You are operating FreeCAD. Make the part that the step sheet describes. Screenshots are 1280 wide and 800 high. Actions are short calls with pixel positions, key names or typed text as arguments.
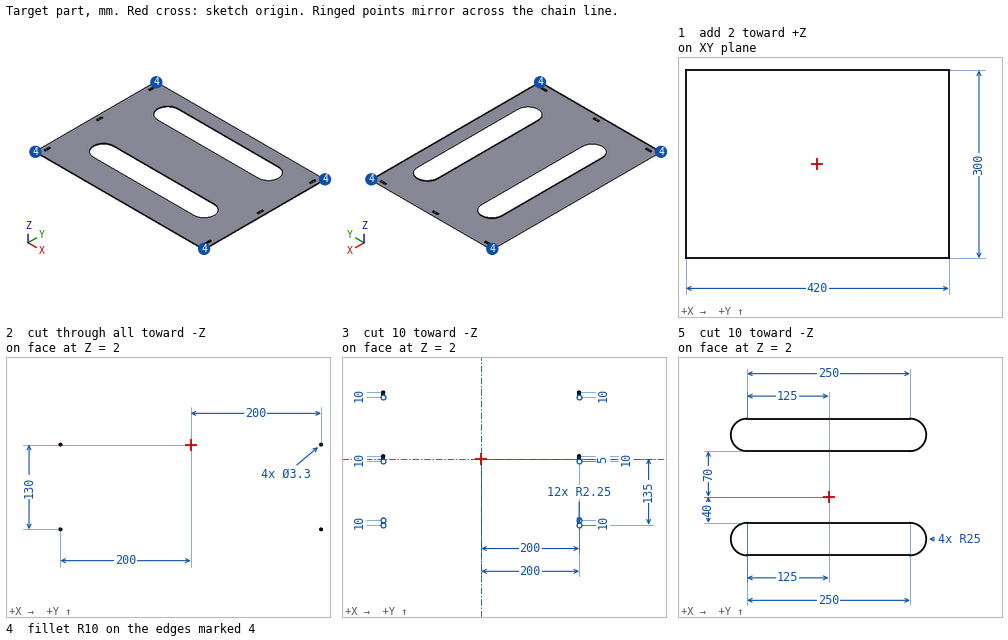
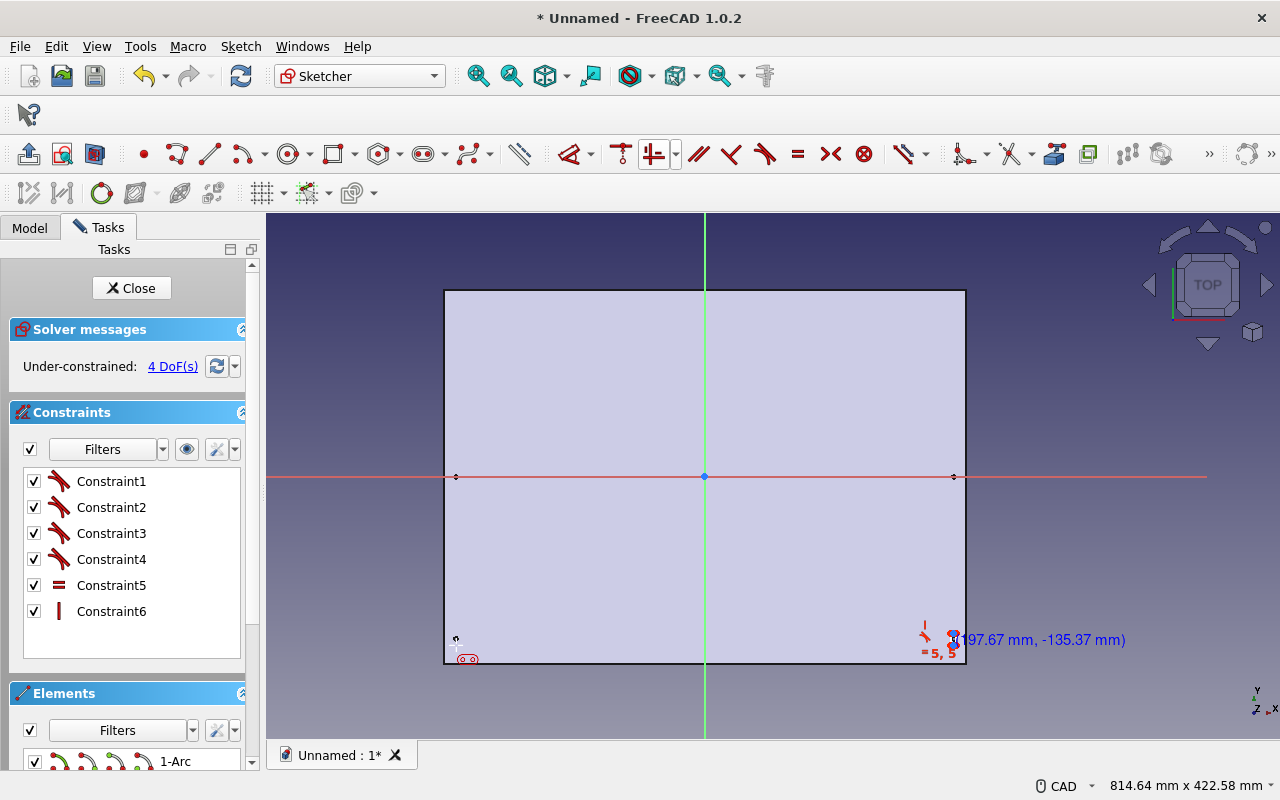
click(456, 645)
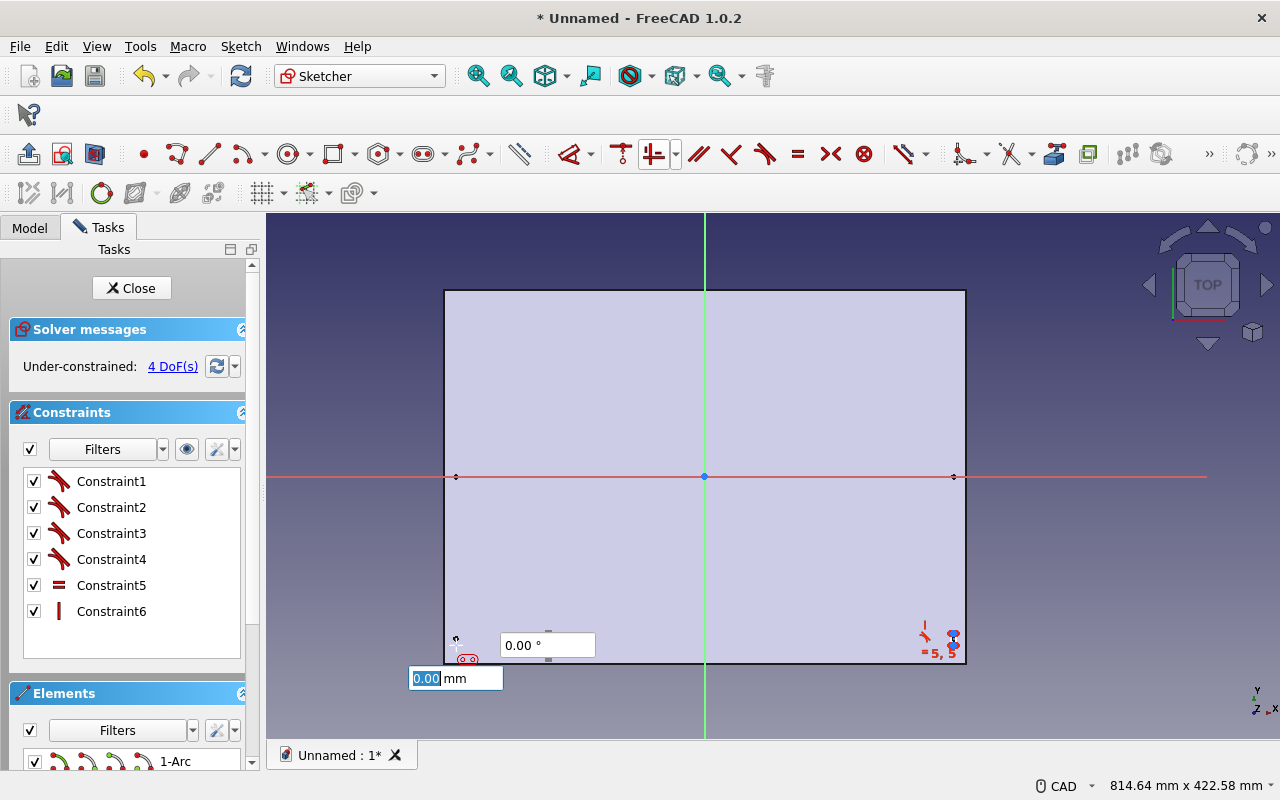
scroll(456, 633, up, 2)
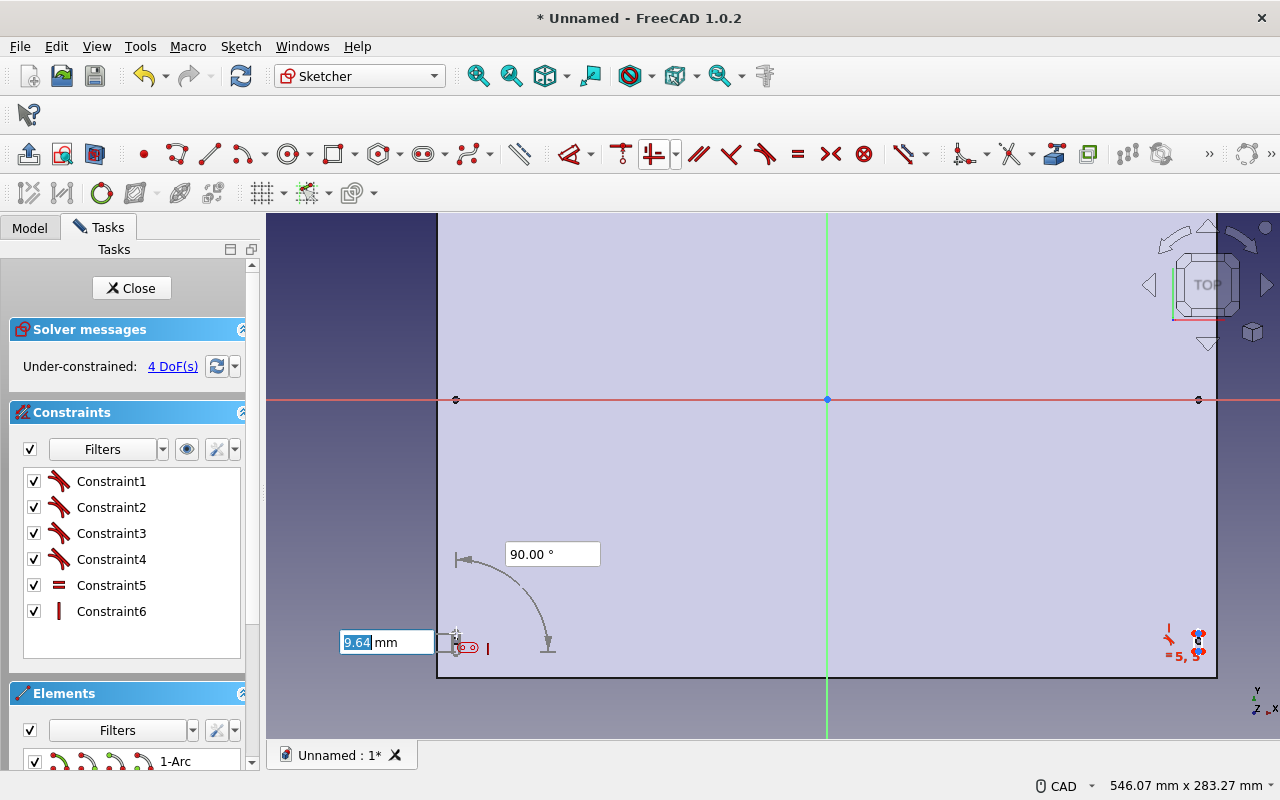
click(456, 632)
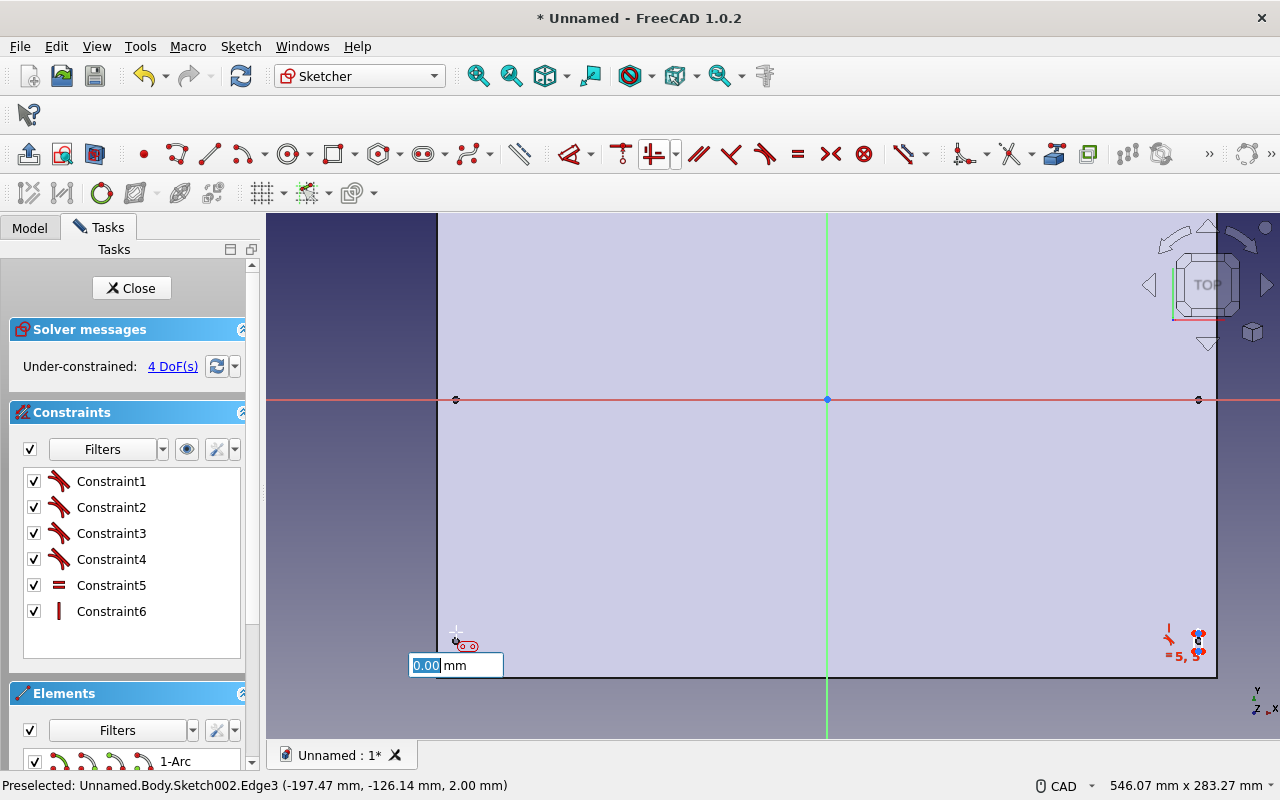
scroll(460, 641, up, 7)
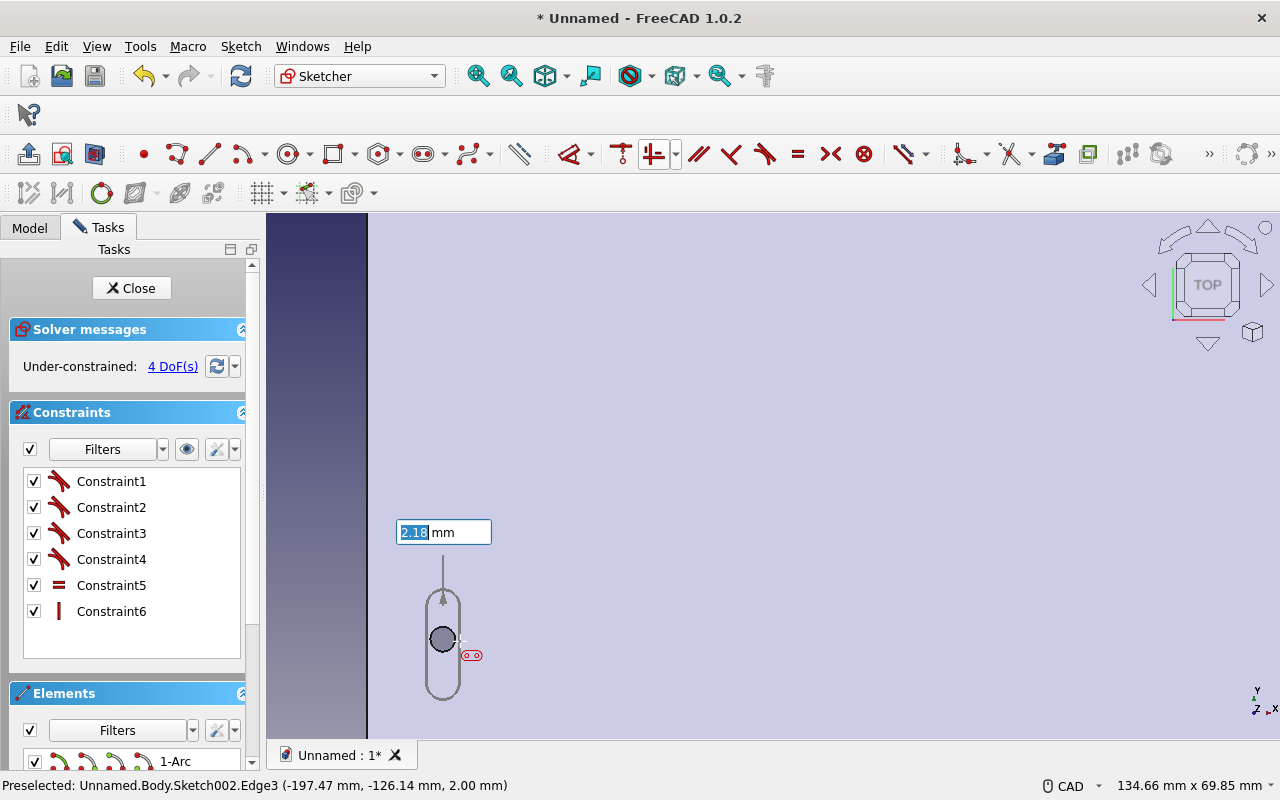
click(460, 639)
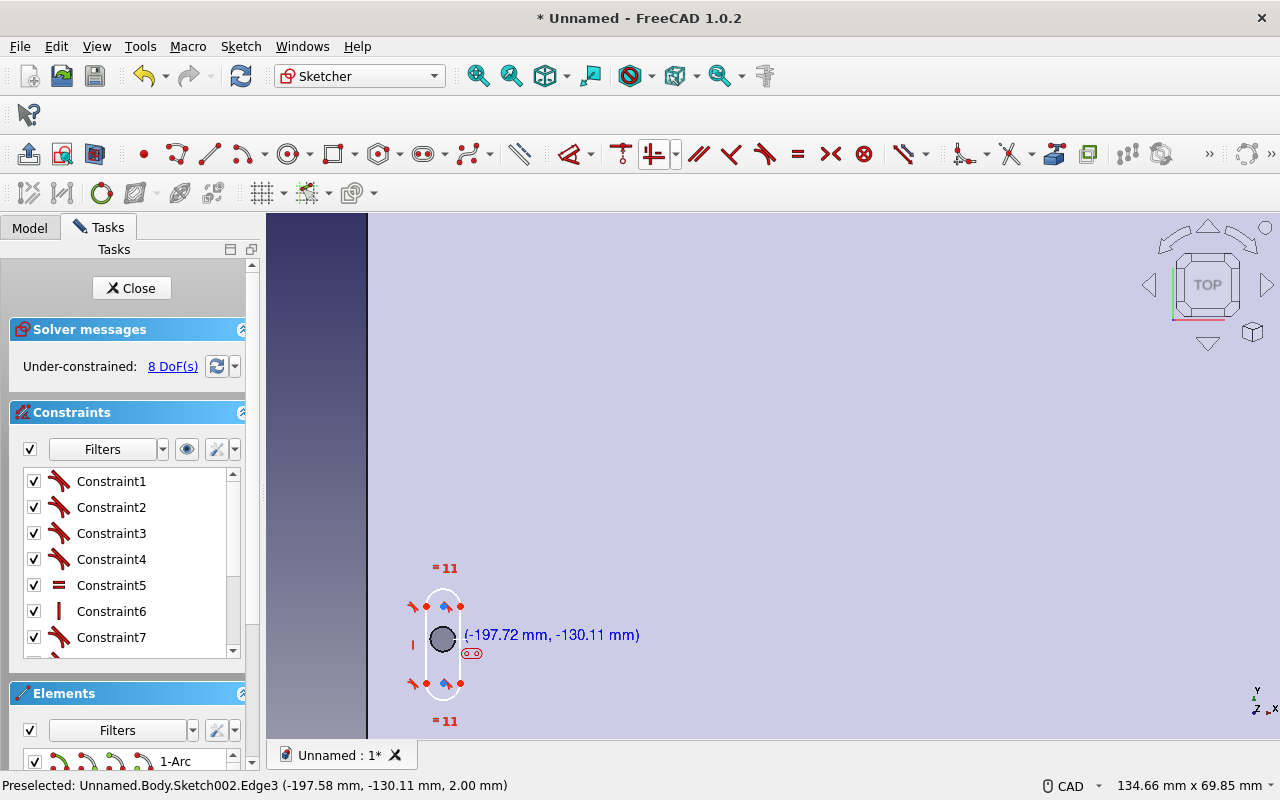
scroll(458, 638, down, 9)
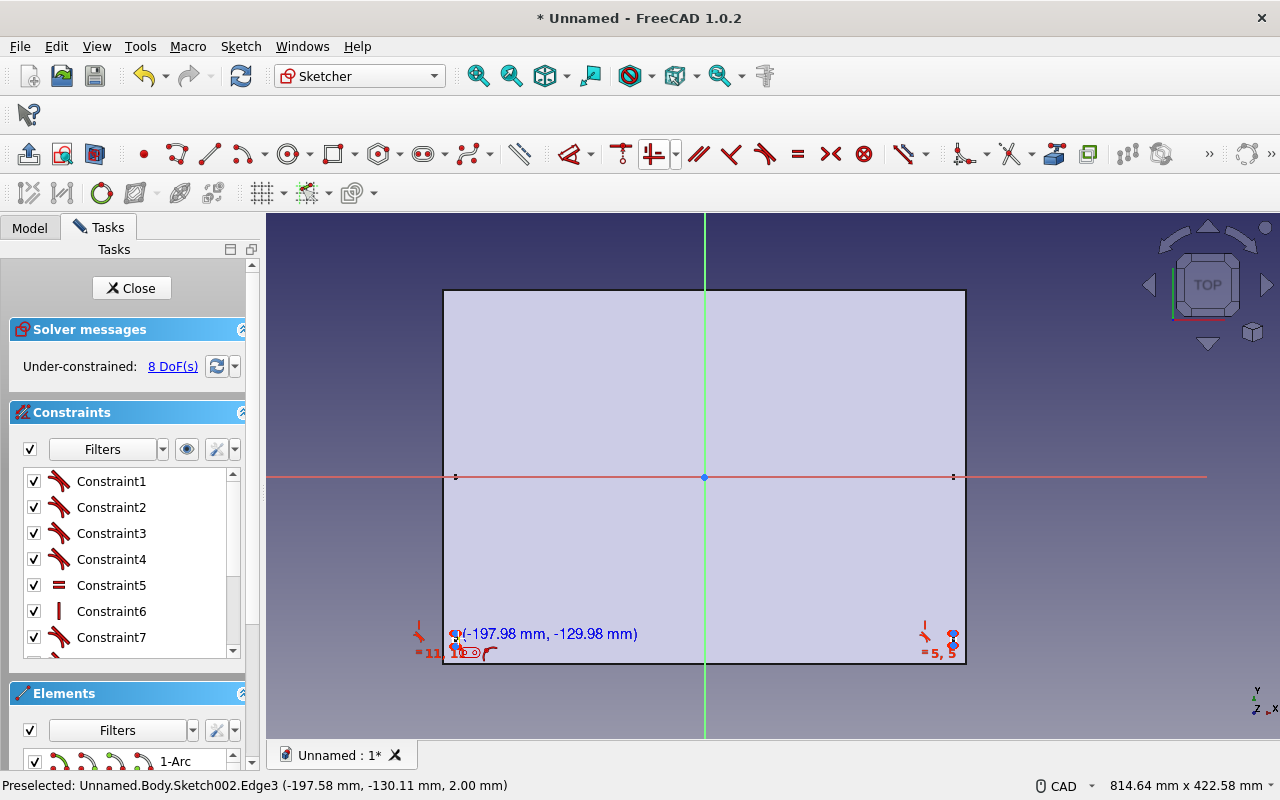
scroll(954, 483, up, 11)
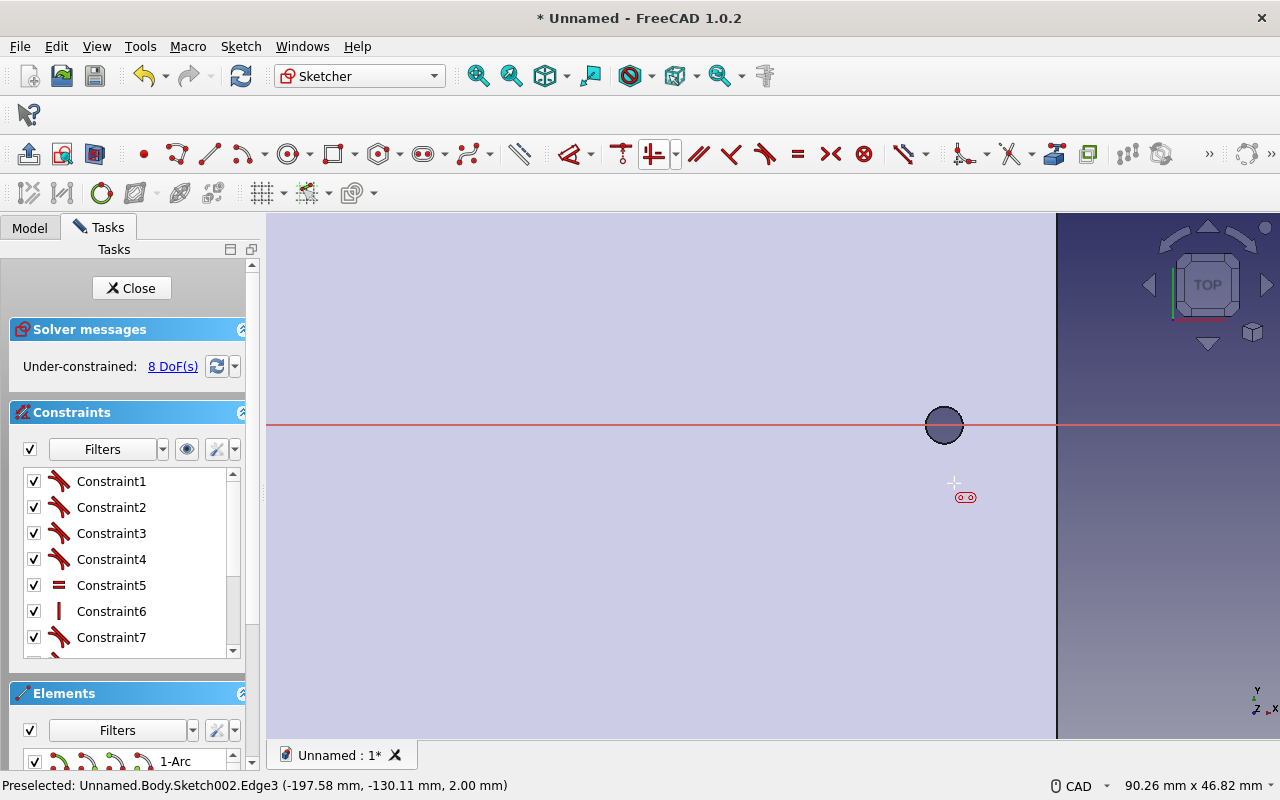
scroll(955, 482, down, 11)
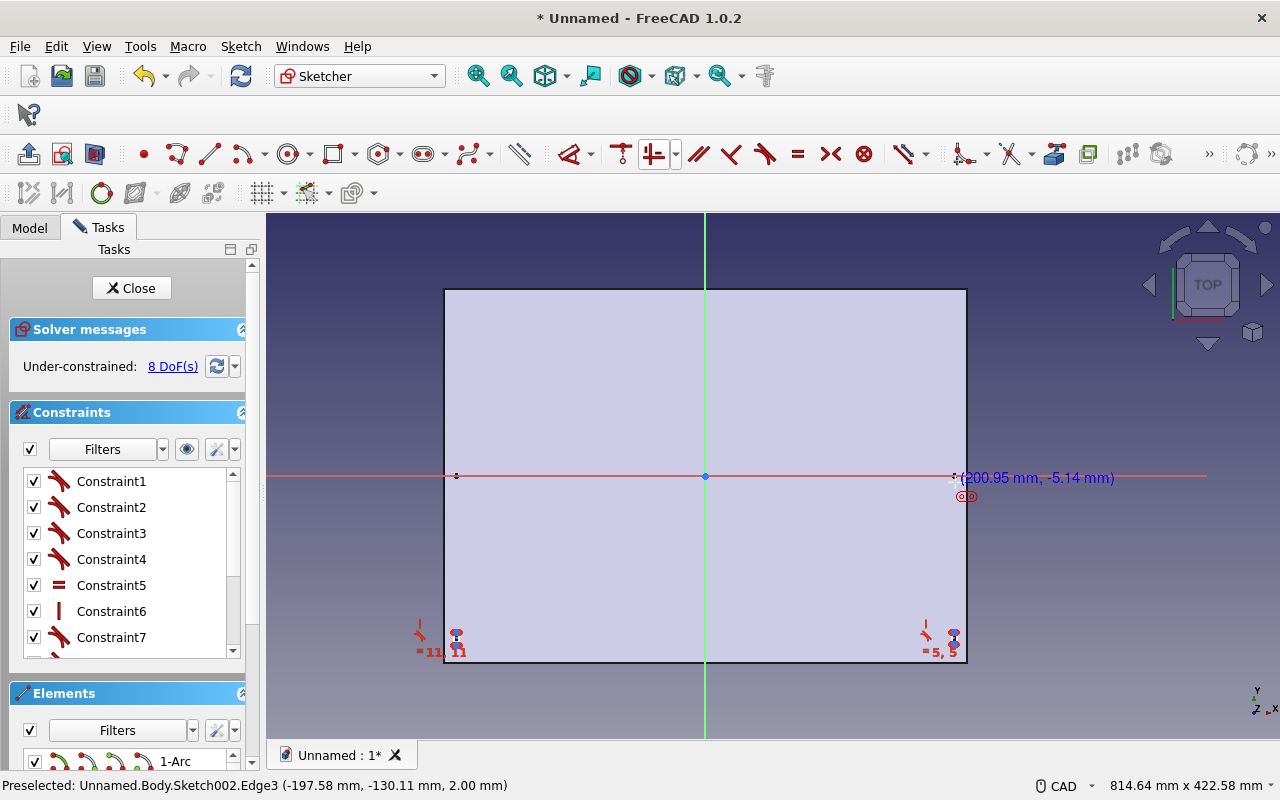
scroll(954, 482, up, 5)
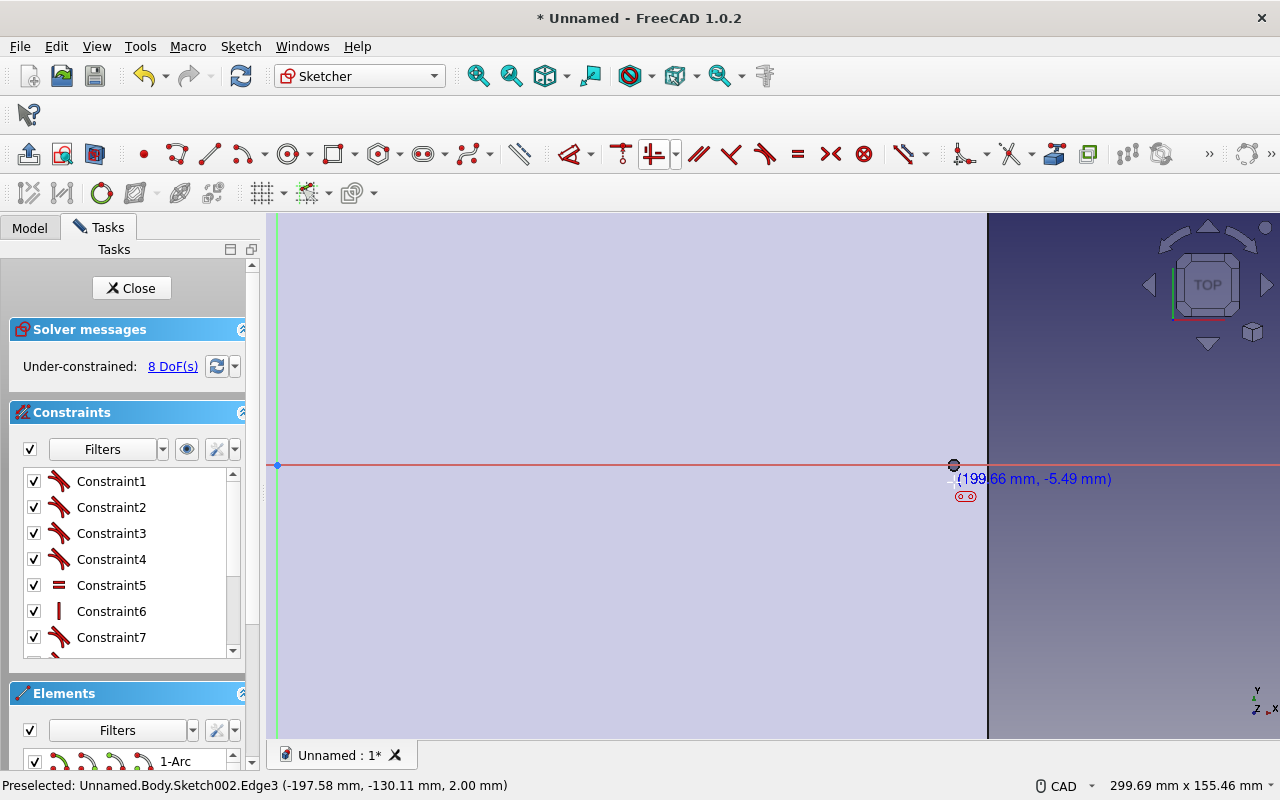
click(954, 482)